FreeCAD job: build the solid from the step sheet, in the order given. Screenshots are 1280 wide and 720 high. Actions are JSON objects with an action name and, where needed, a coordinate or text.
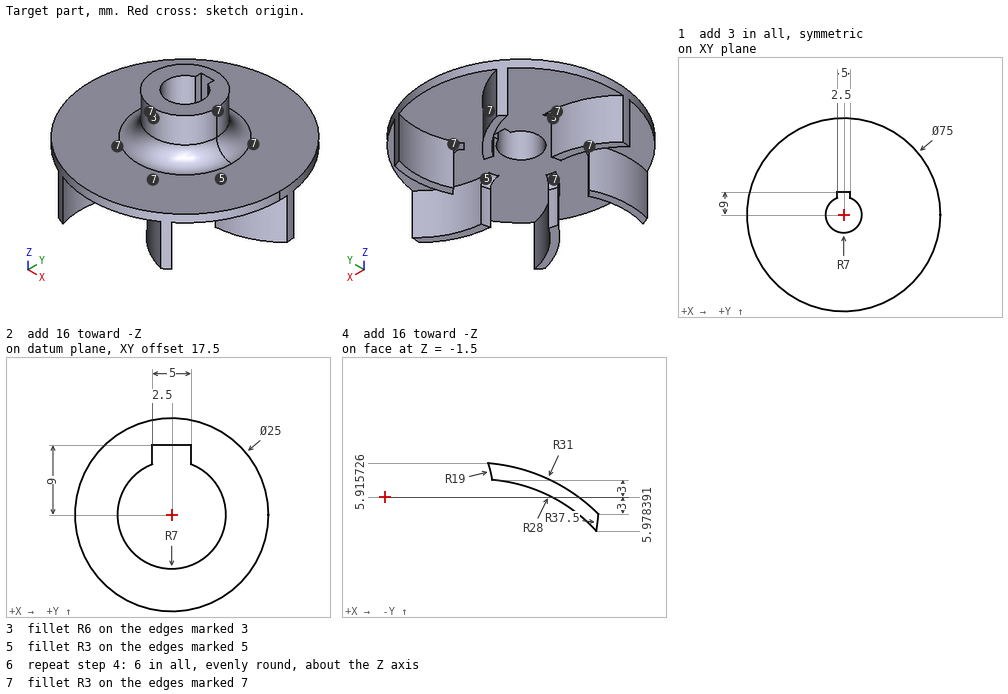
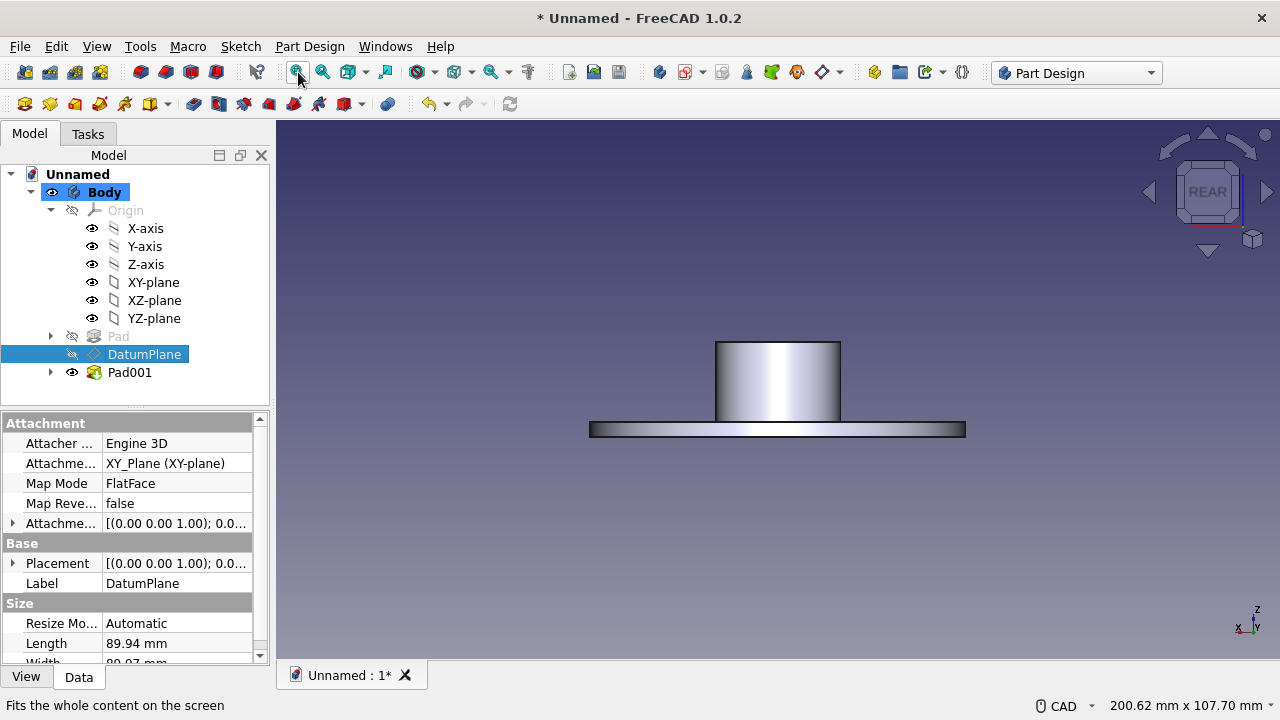
{"action": "key", "text": "6"}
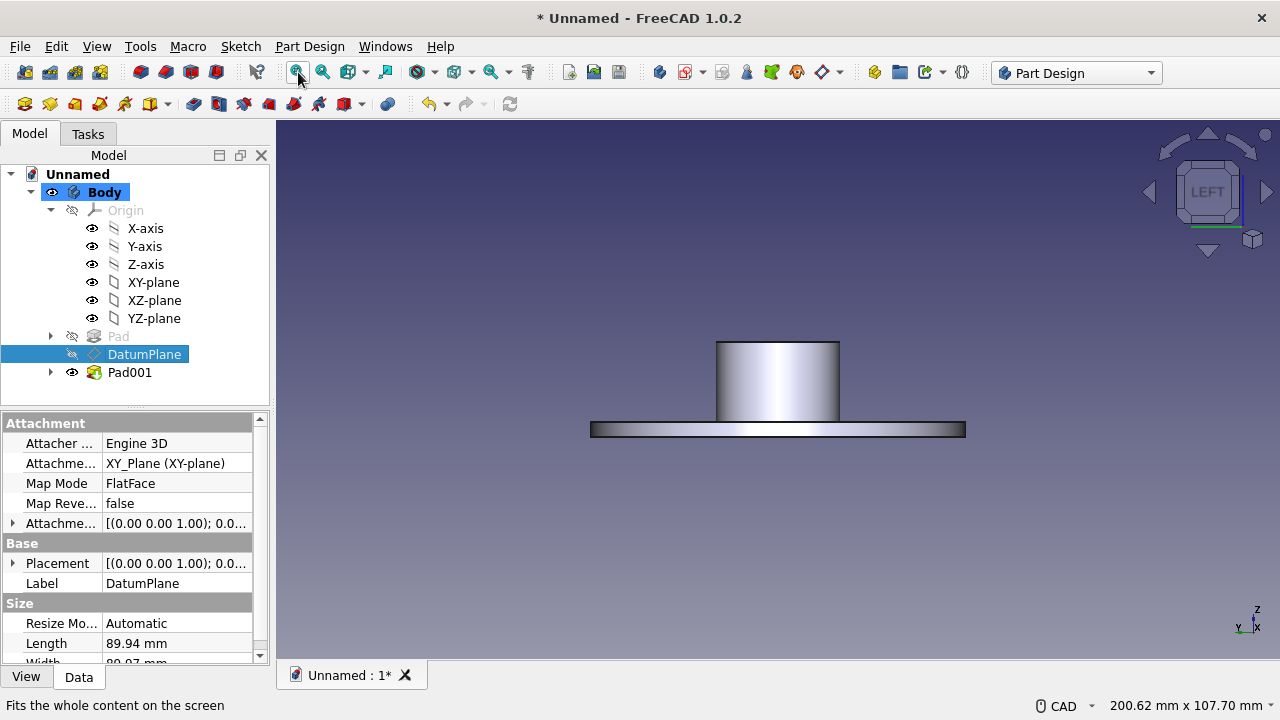
{"action": "left_click", "coordinate": [298, 72]}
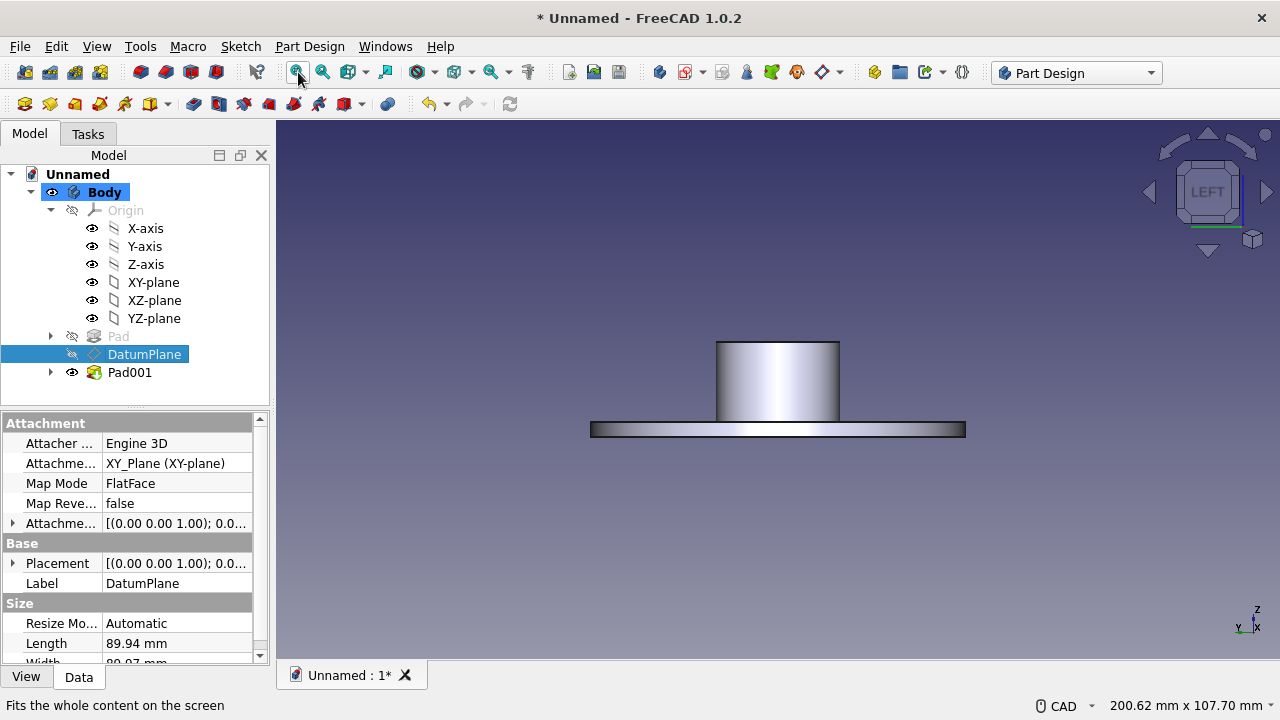
{"action": "key", "text": "v 3"}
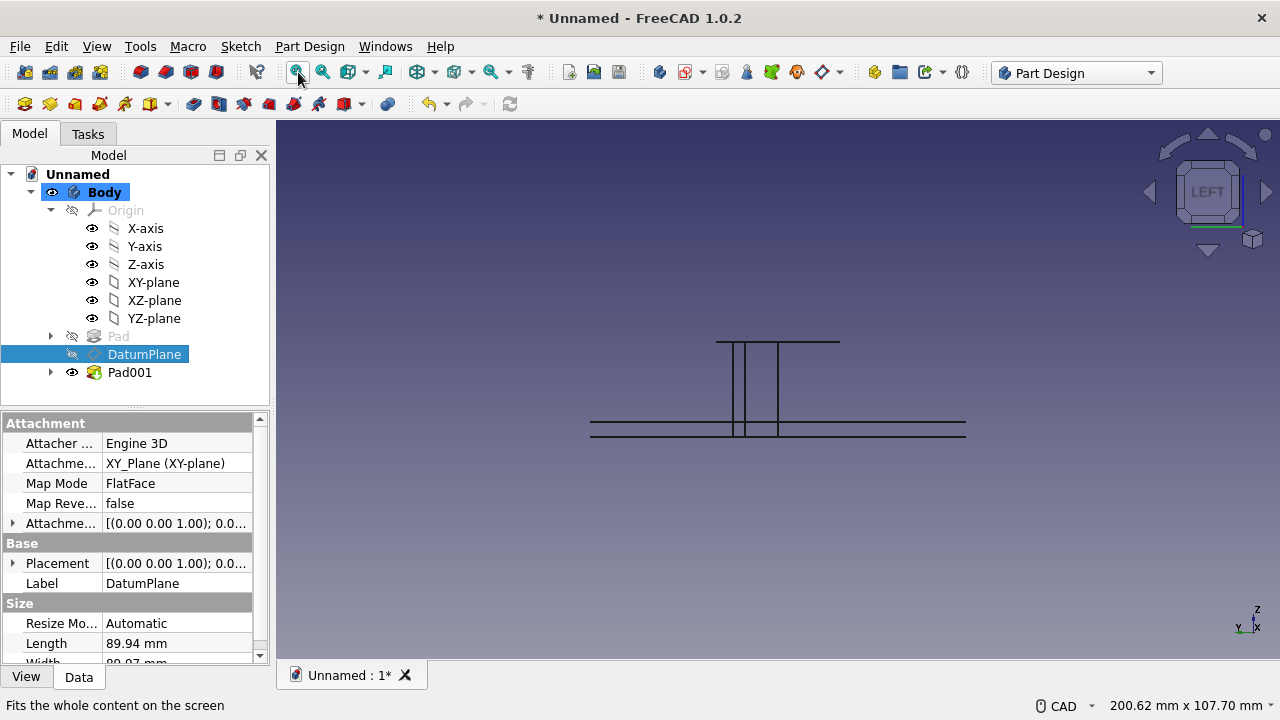
{"action": "key", "text": "0"}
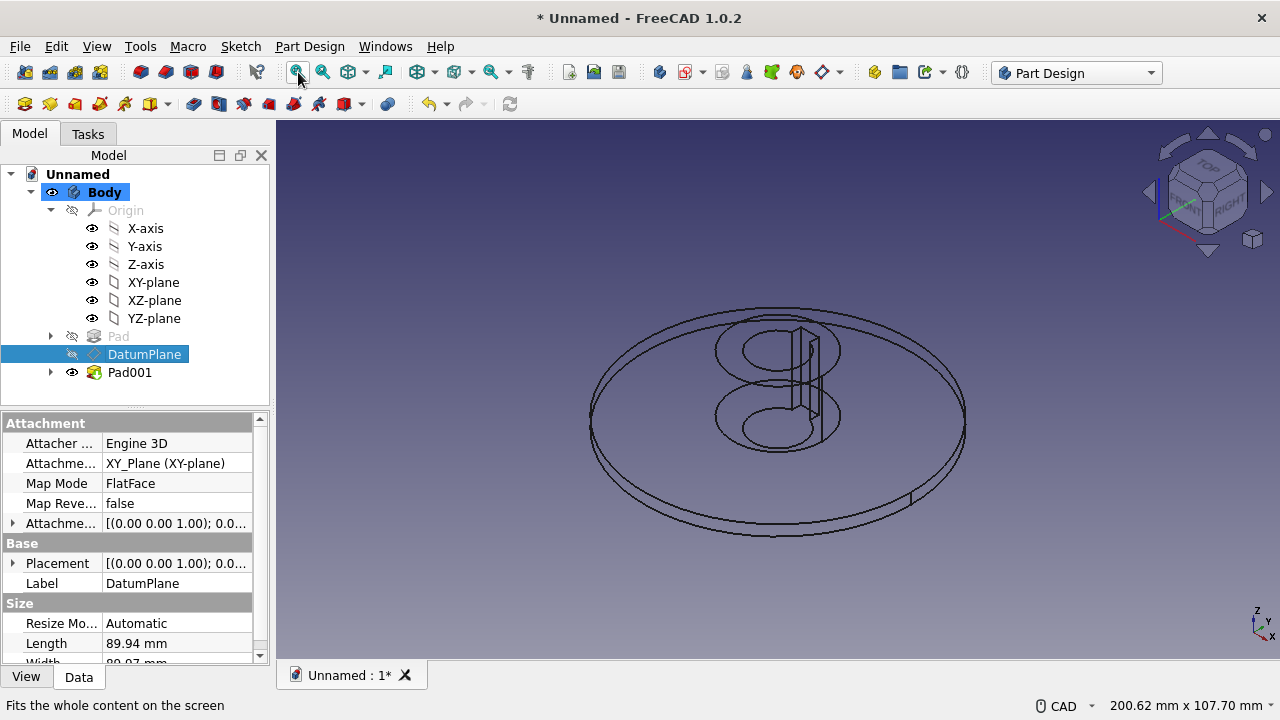
{"action": "left_click", "coordinate": [734, 389]}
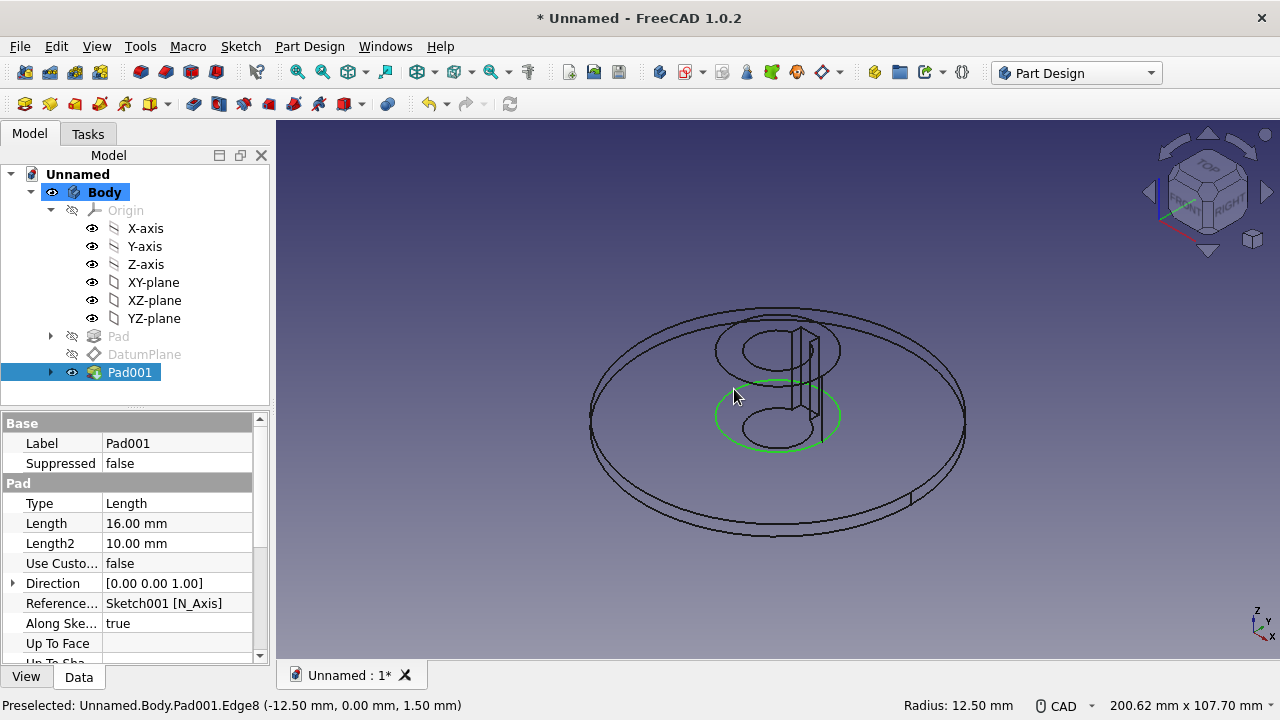
{"action": "key", "text": "v 1"}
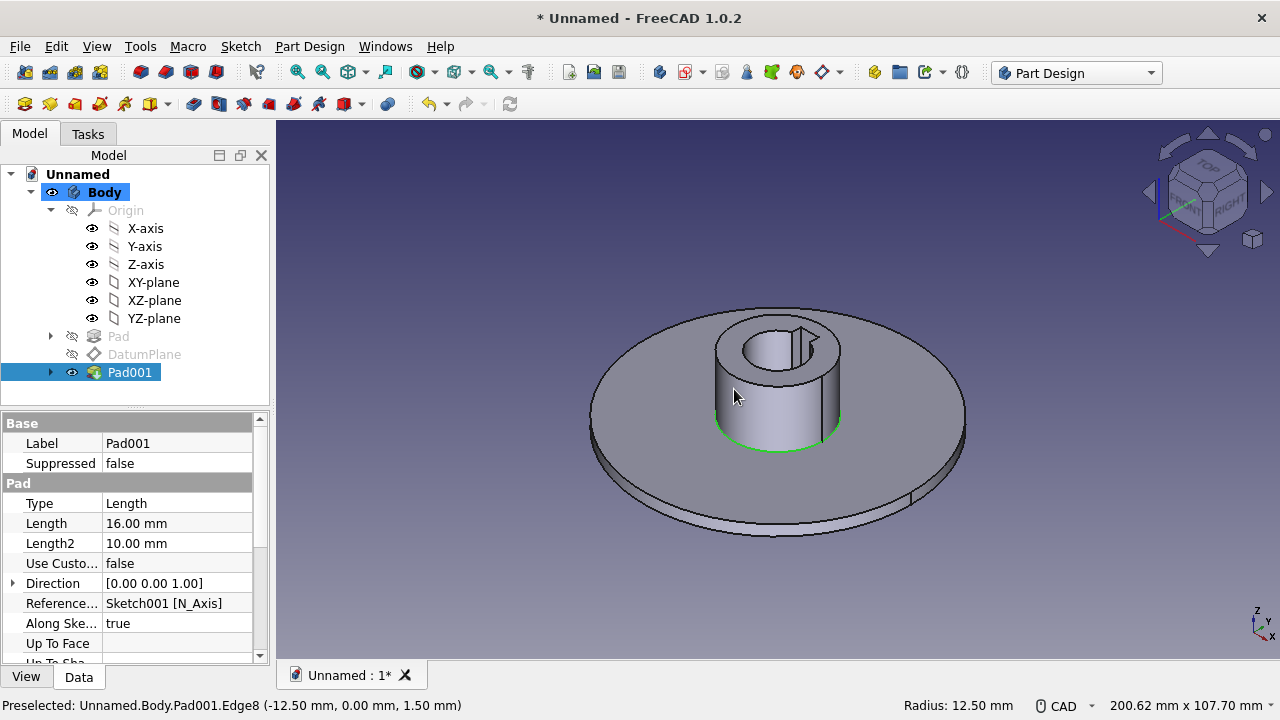
{"action": "left_click", "coordinate": [141, 72]}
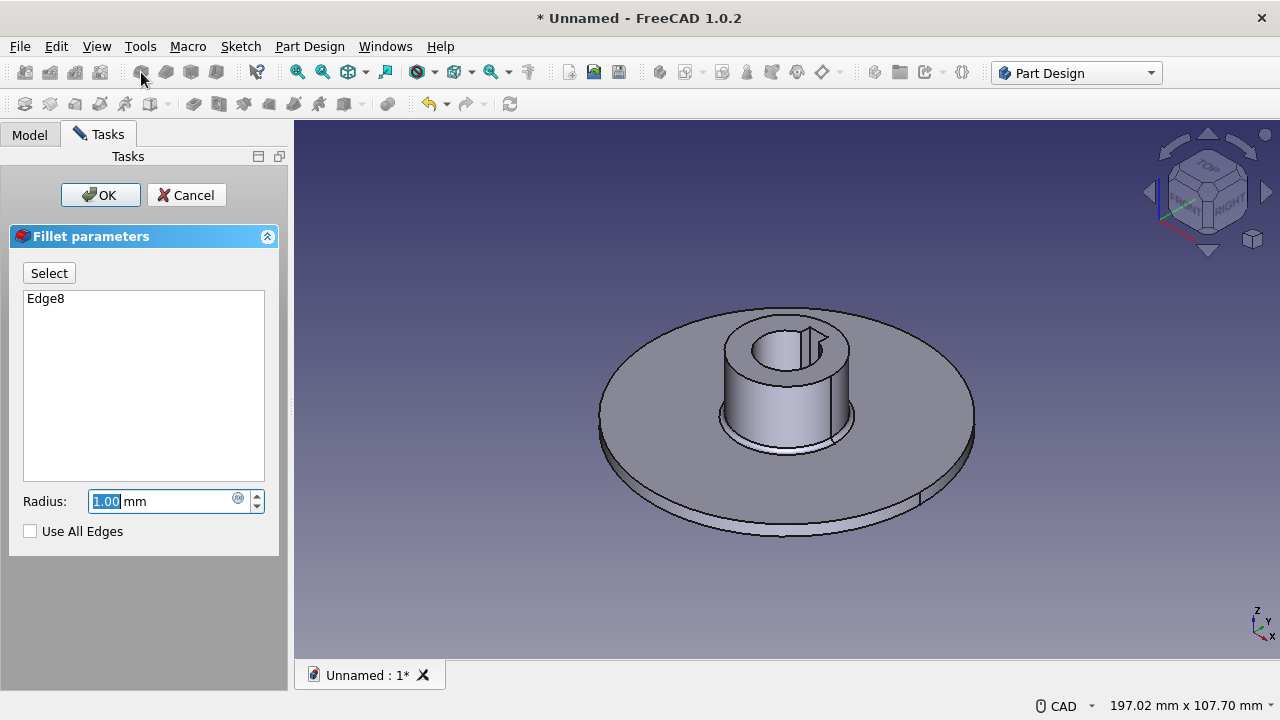
{"action": "type", "text": "6"}
{"action": "key", "text": "Tab"}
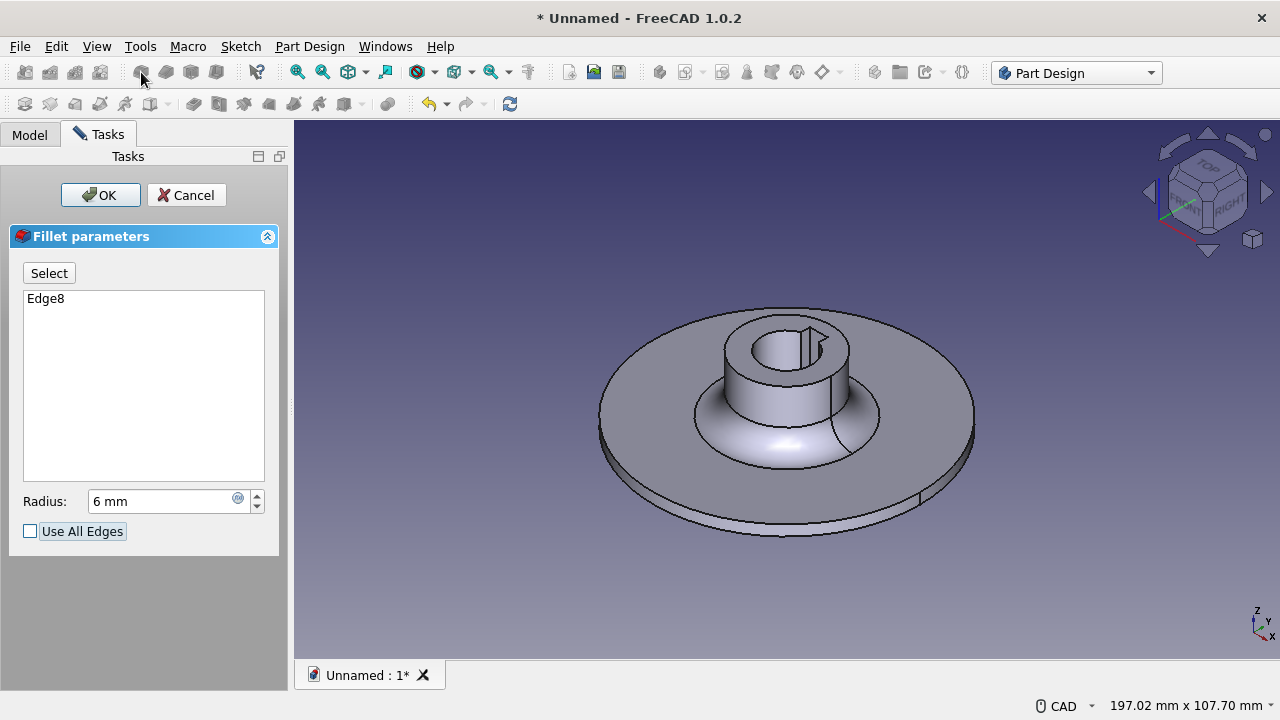
{"action": "left_click", "coordinate": [101, 195]}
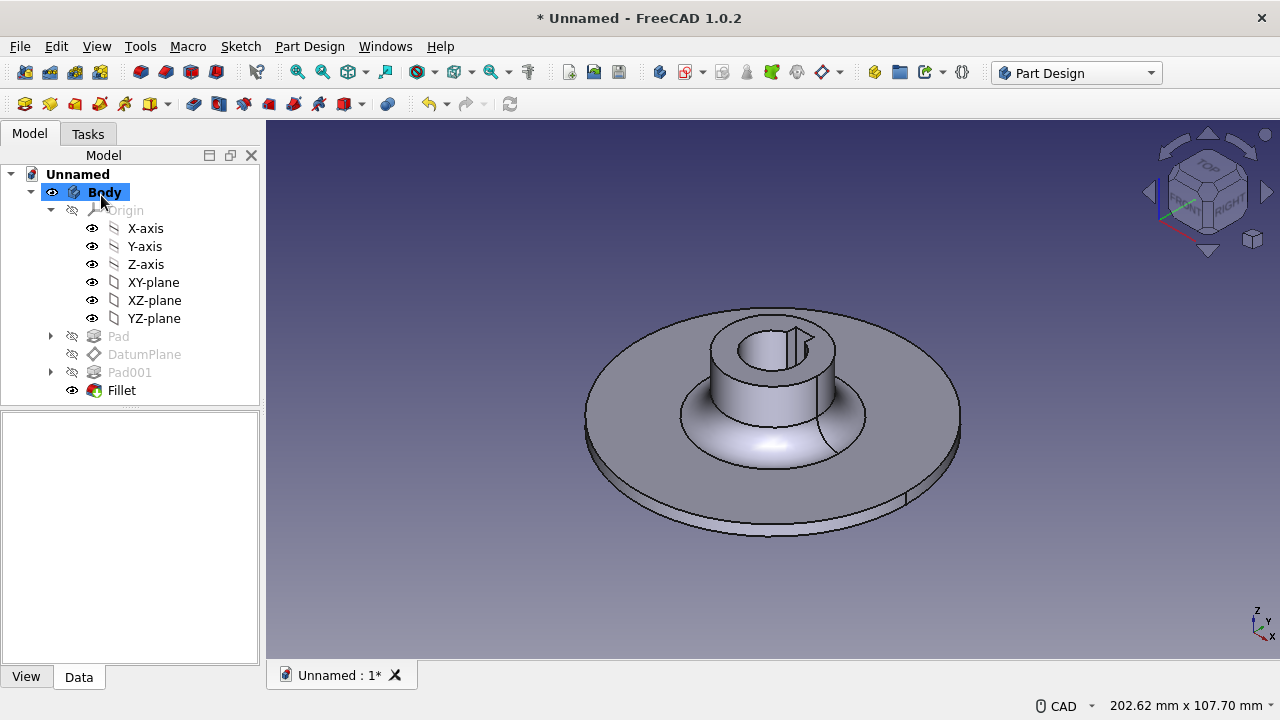
{"action": "key", "text": "5"}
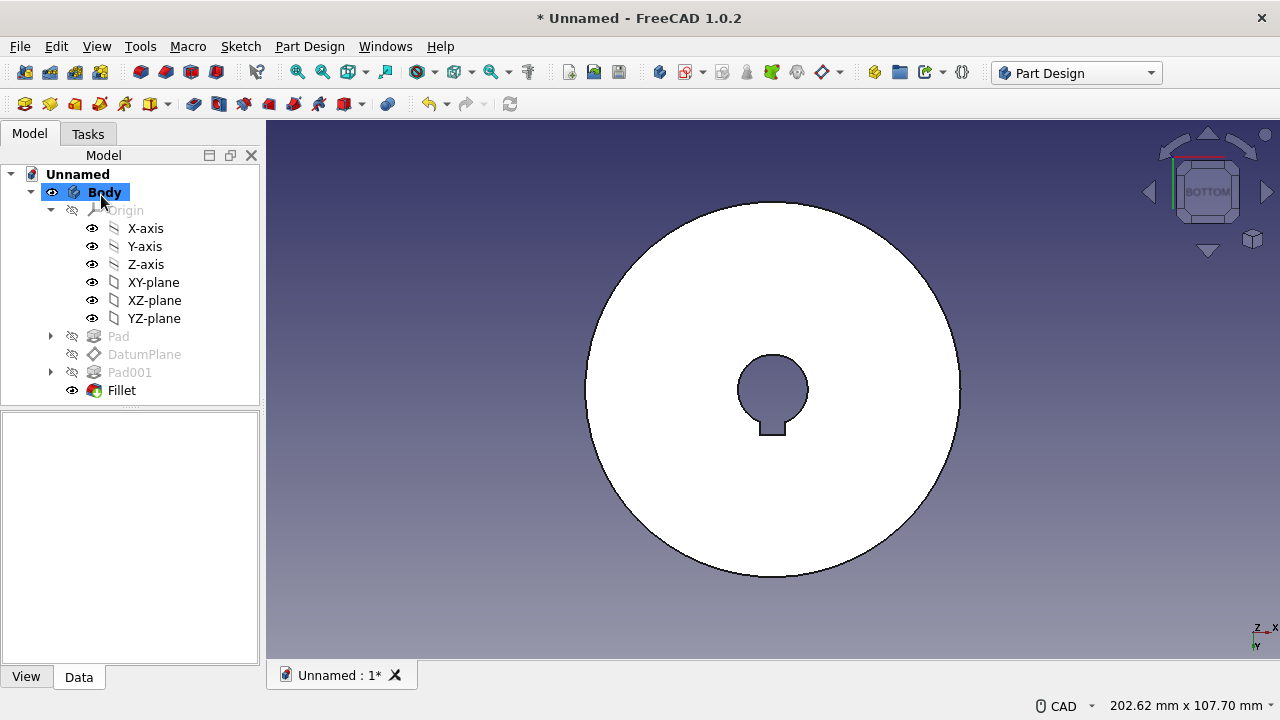
{"action": "left_click", "coordinate": [666, 388]}